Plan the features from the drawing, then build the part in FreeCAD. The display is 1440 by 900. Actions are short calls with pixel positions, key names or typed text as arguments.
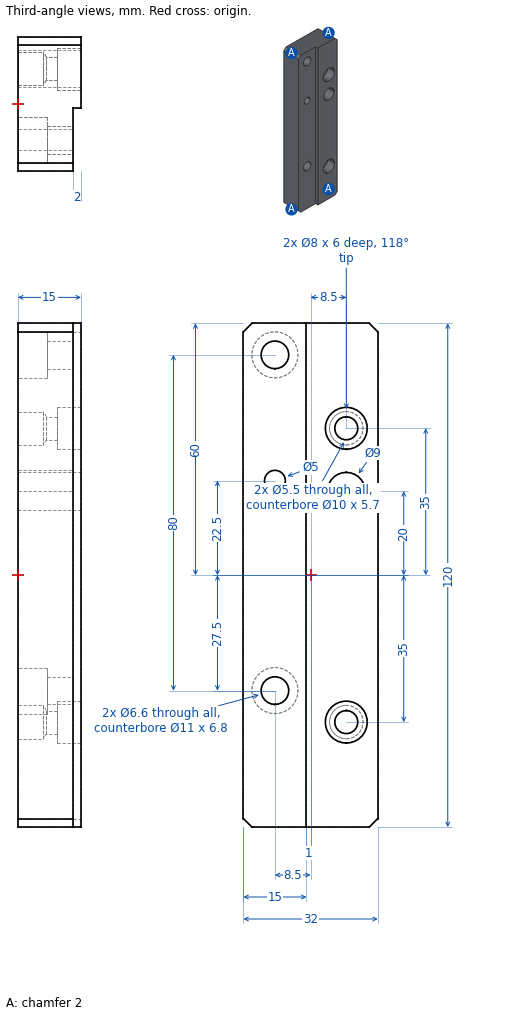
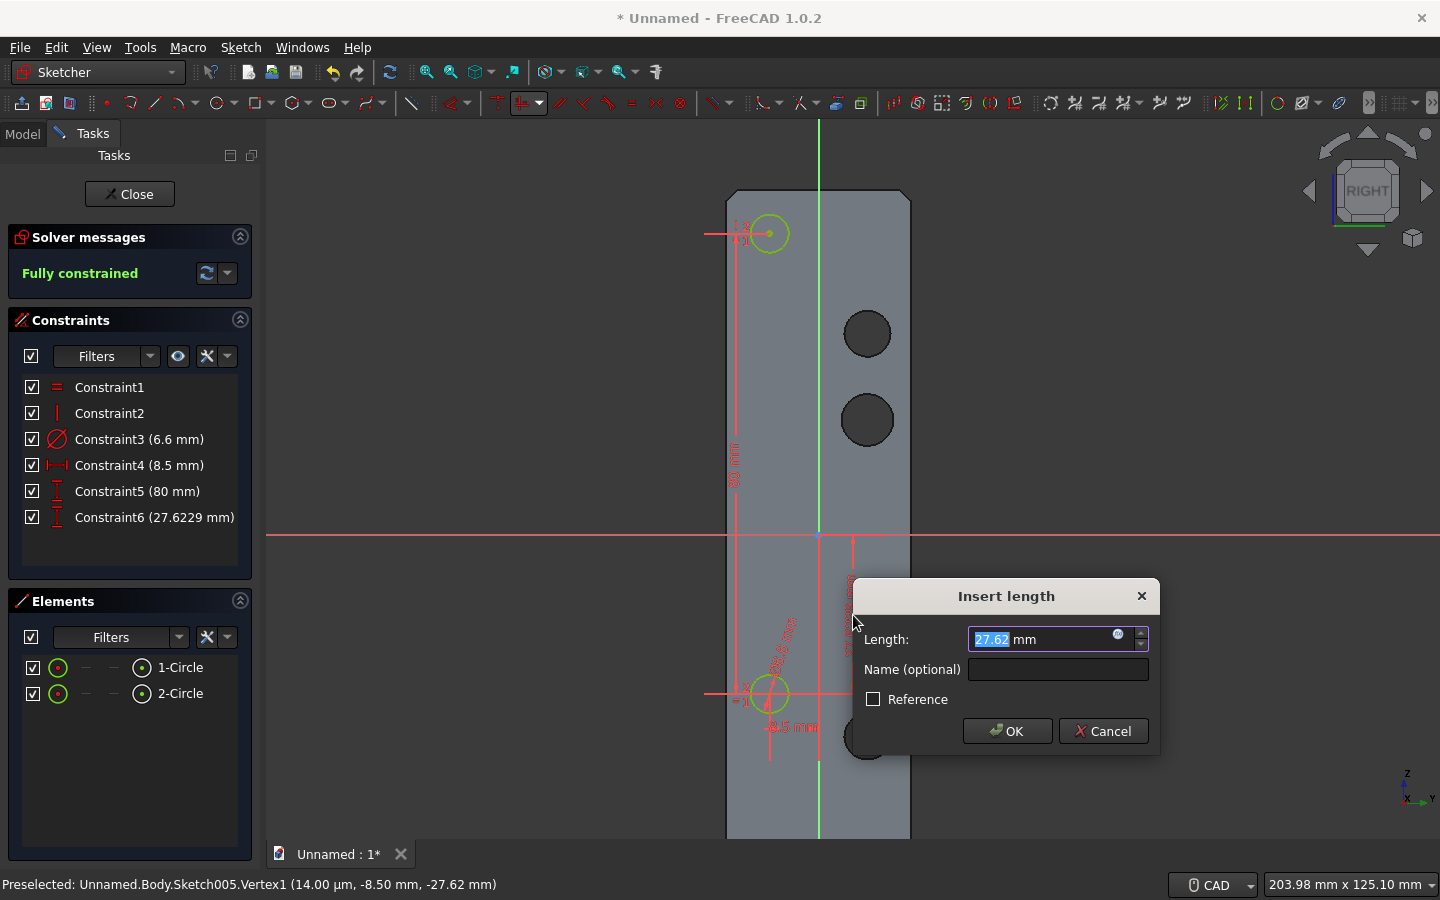
text(27.5)
key(Return)
key(Escape)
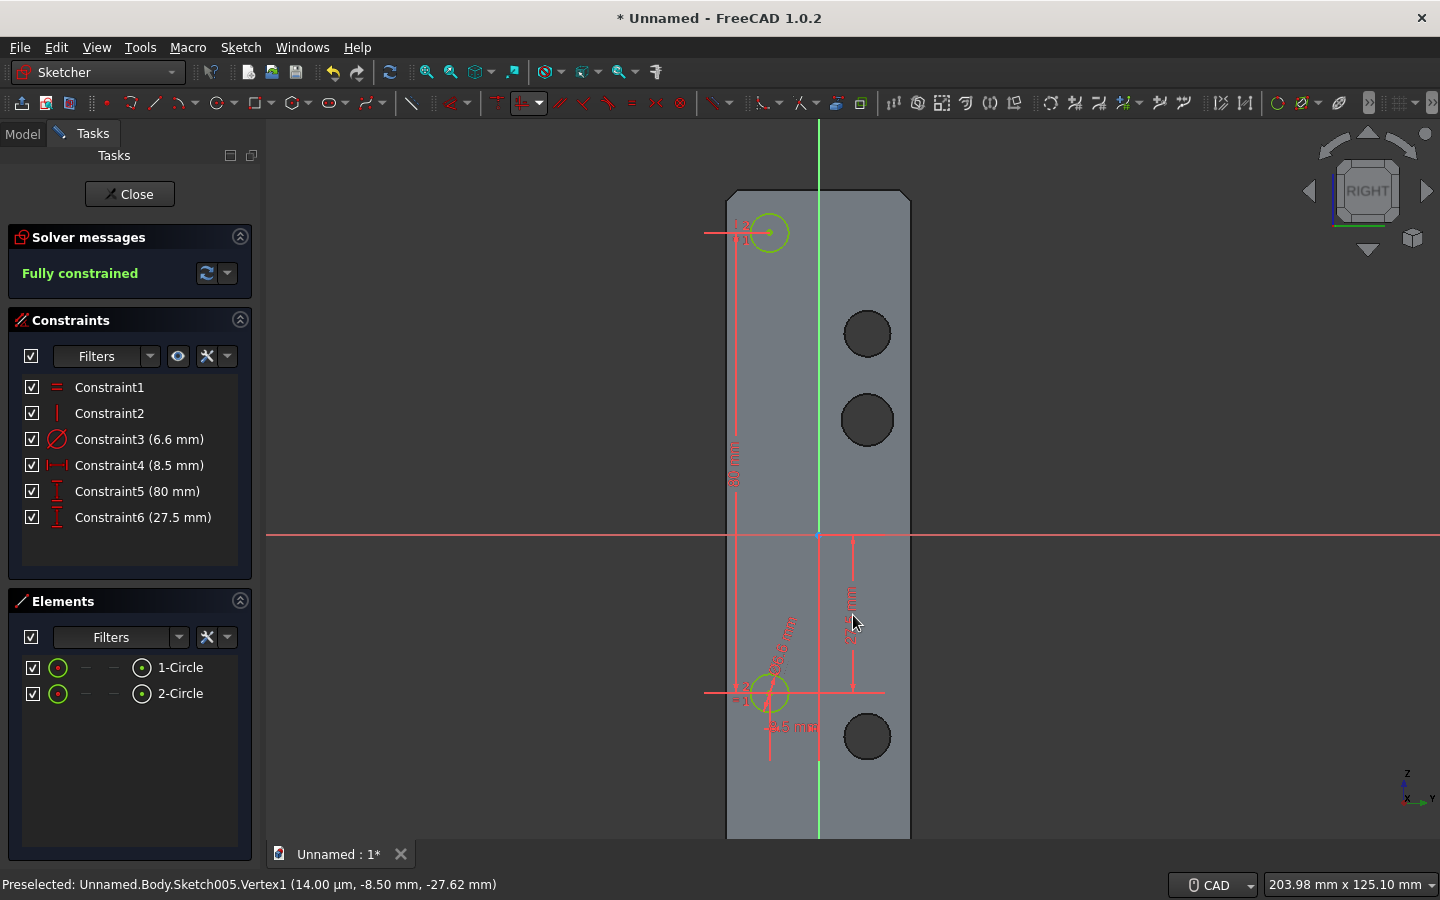
click(130, 194)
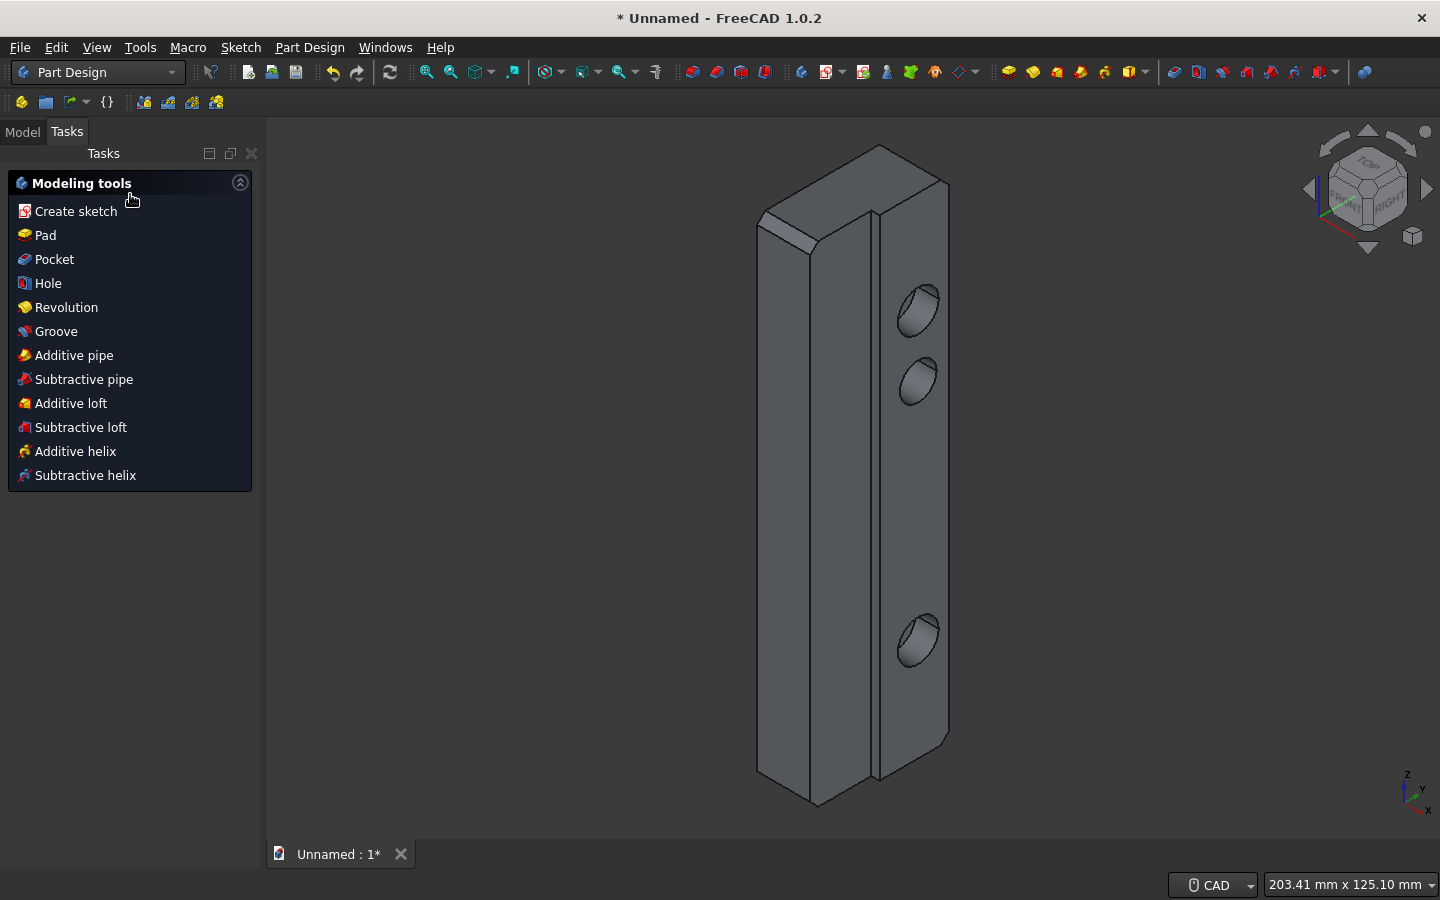
click(1200, 72)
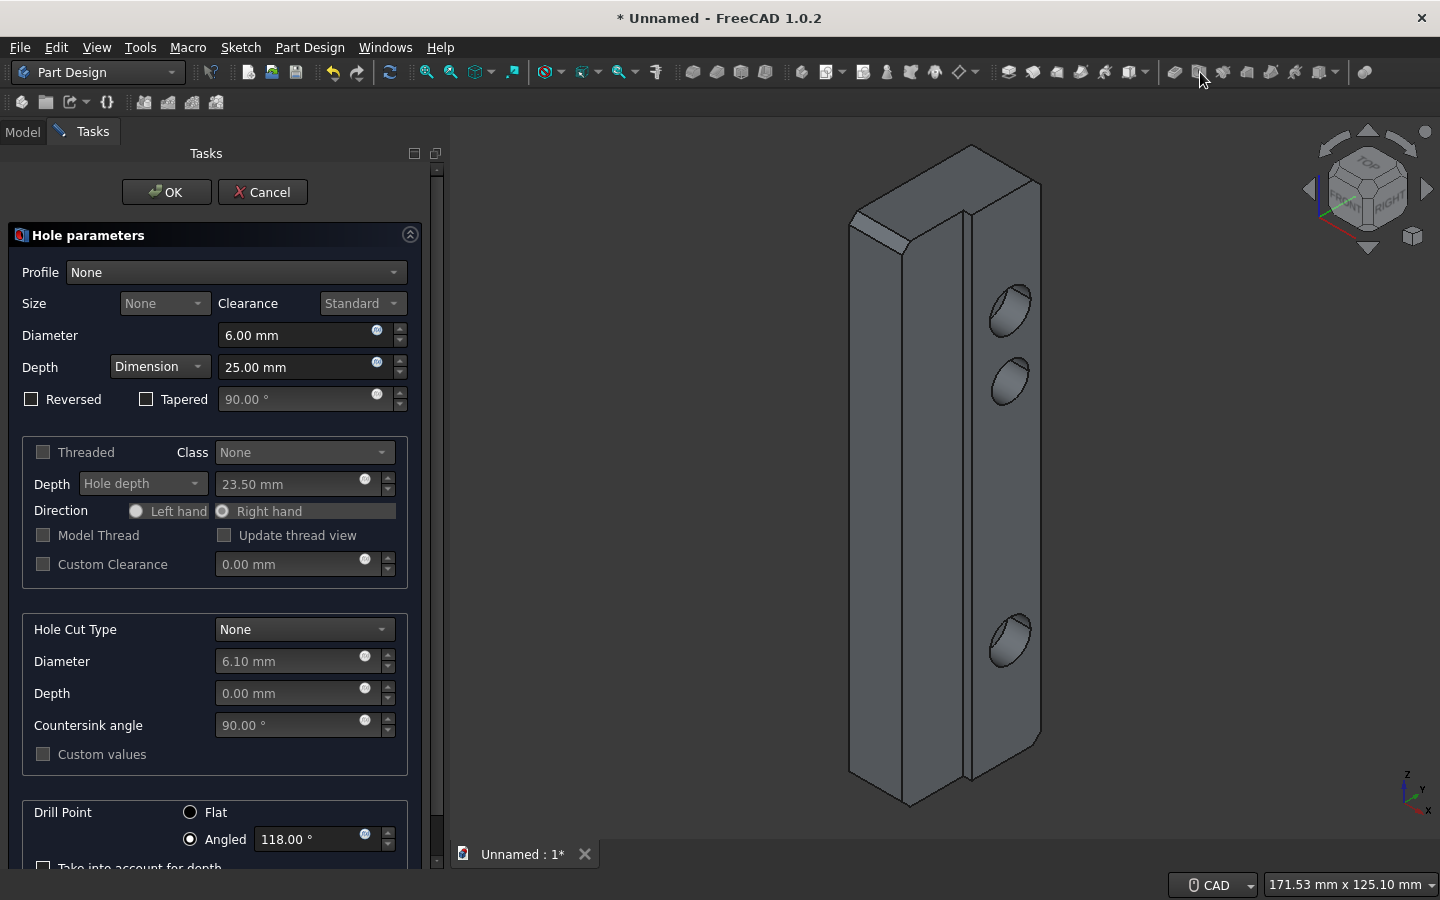
triple_click(305, 335)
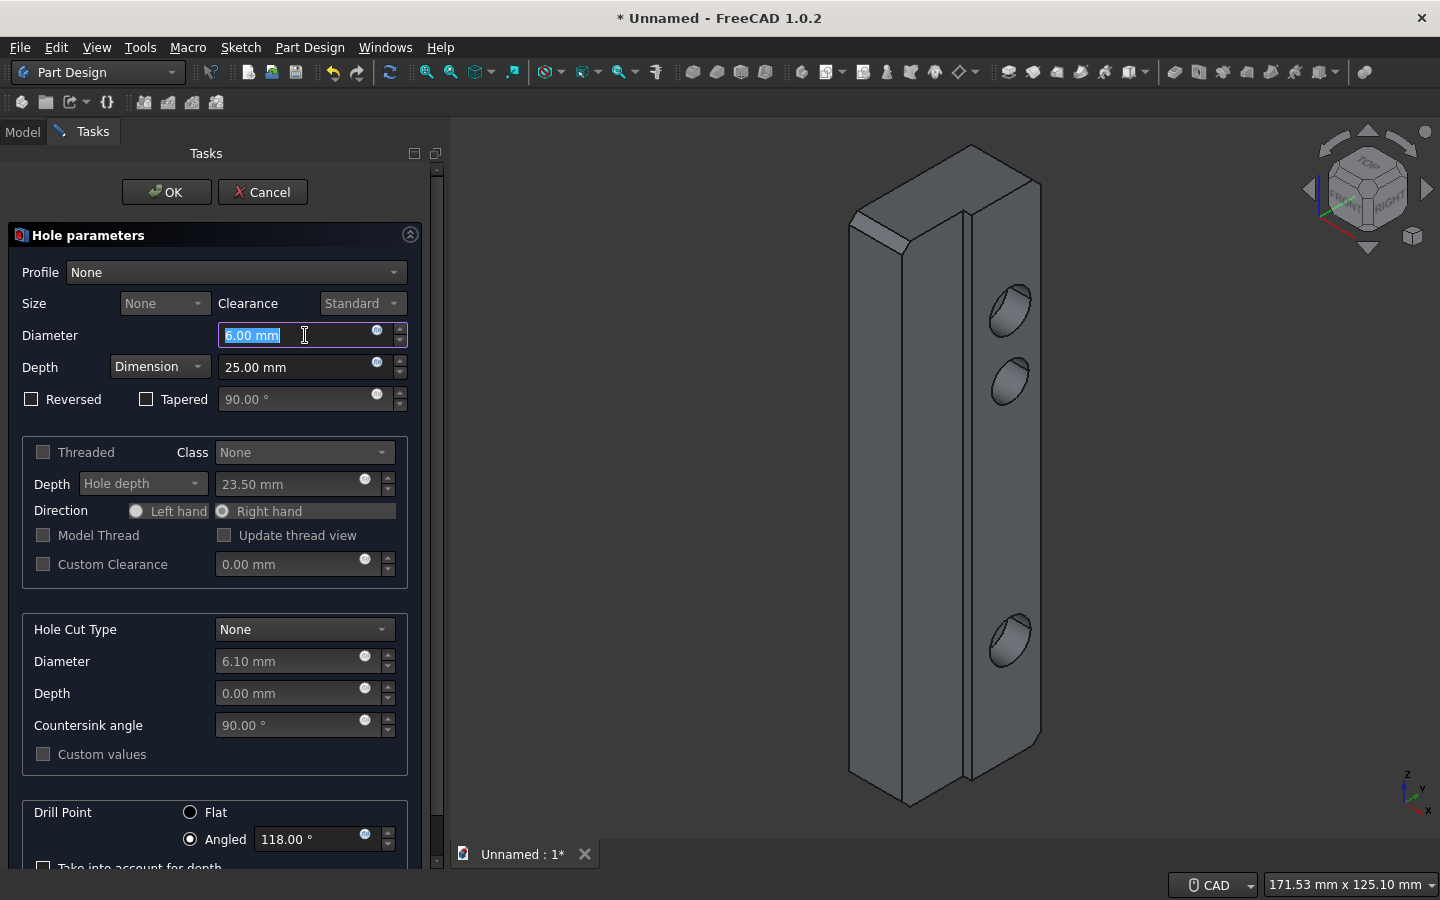
text(6.6)
key(Tab)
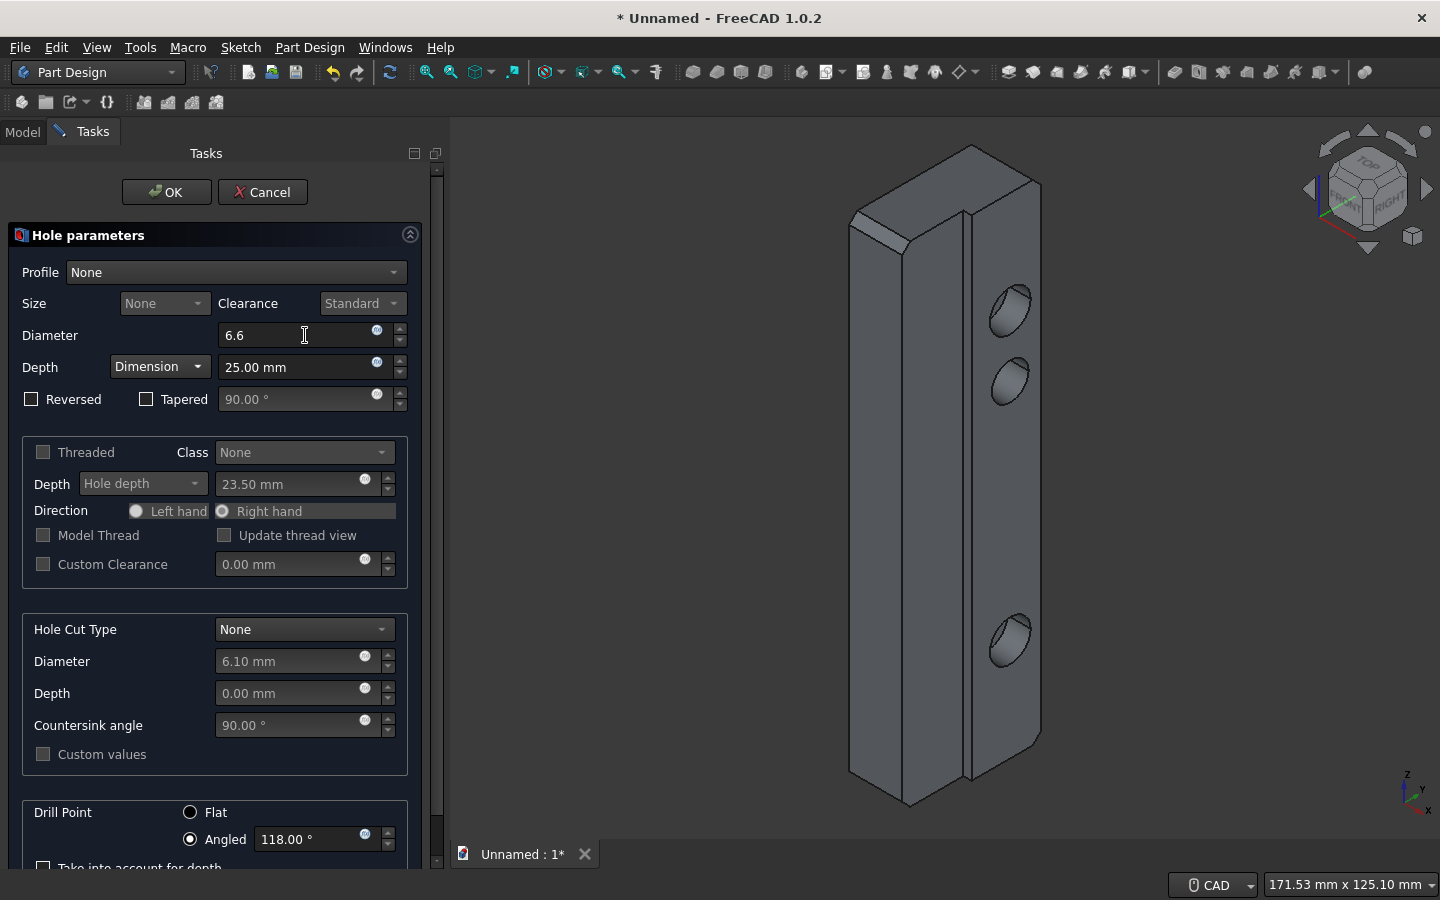
click(161, 366)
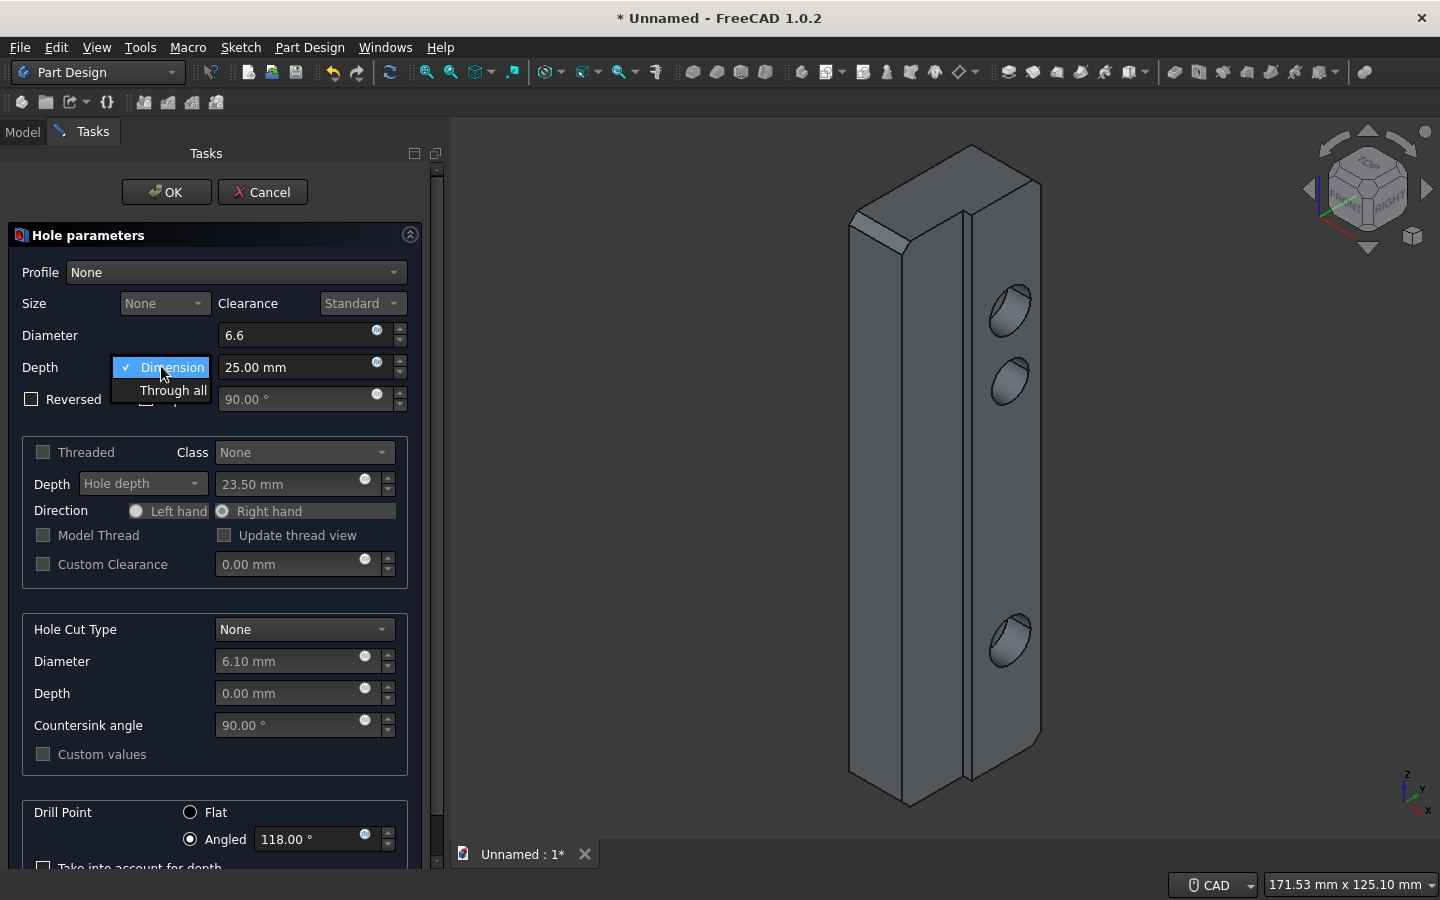
click(160, 390)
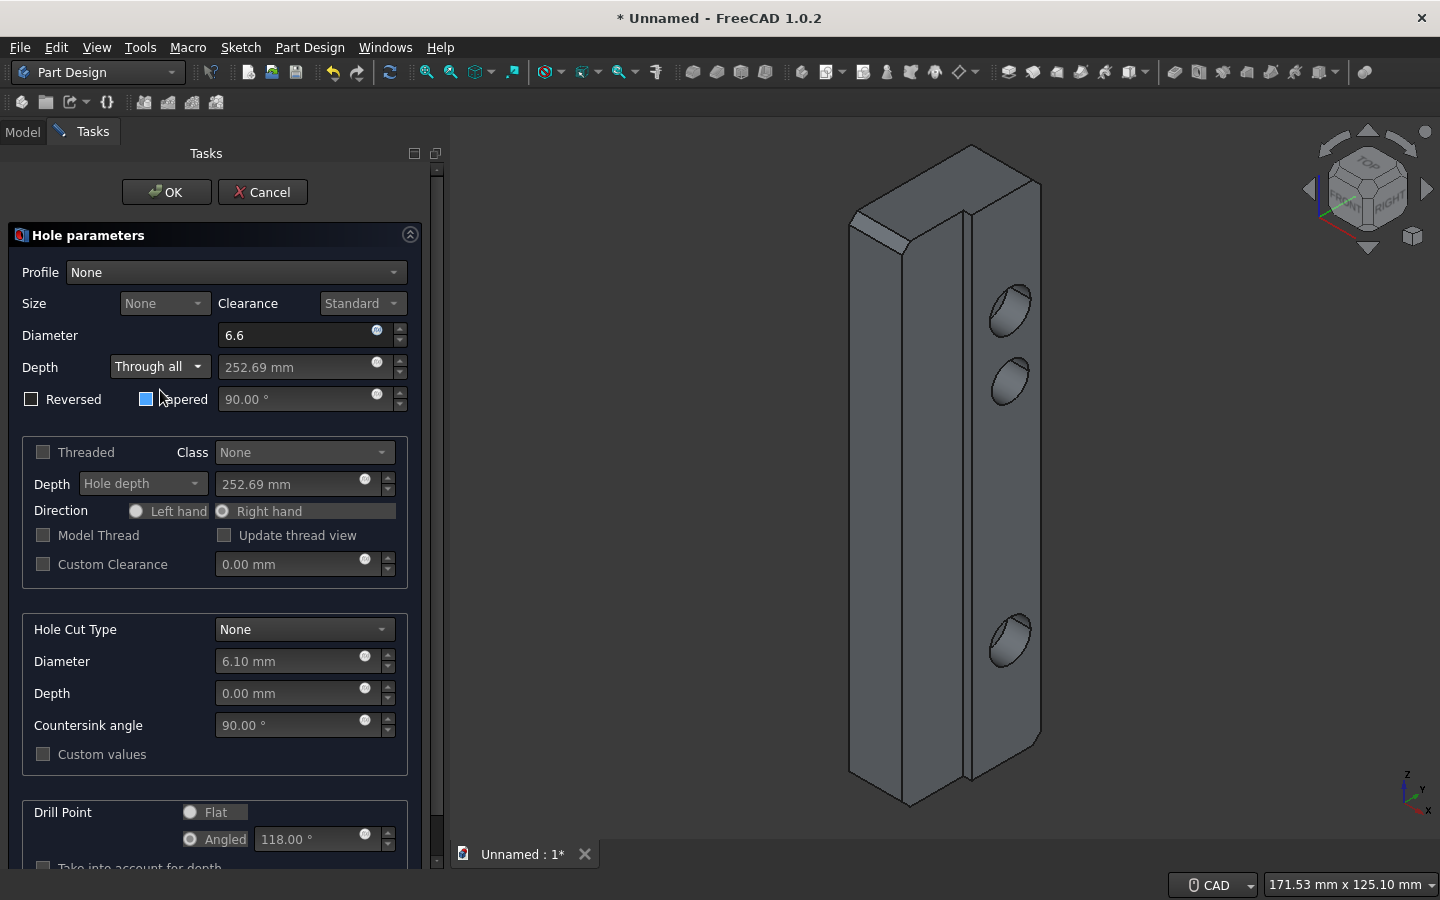
click(30, 399)